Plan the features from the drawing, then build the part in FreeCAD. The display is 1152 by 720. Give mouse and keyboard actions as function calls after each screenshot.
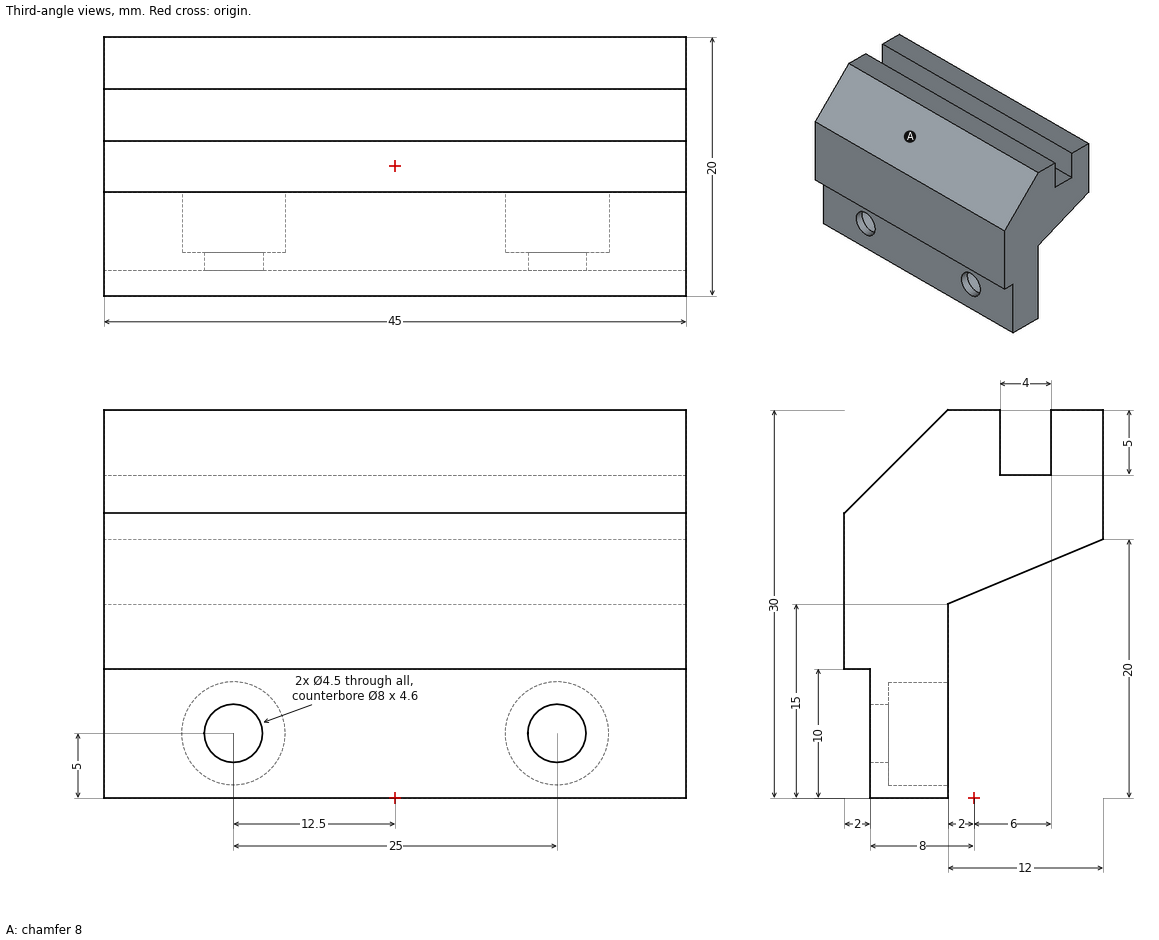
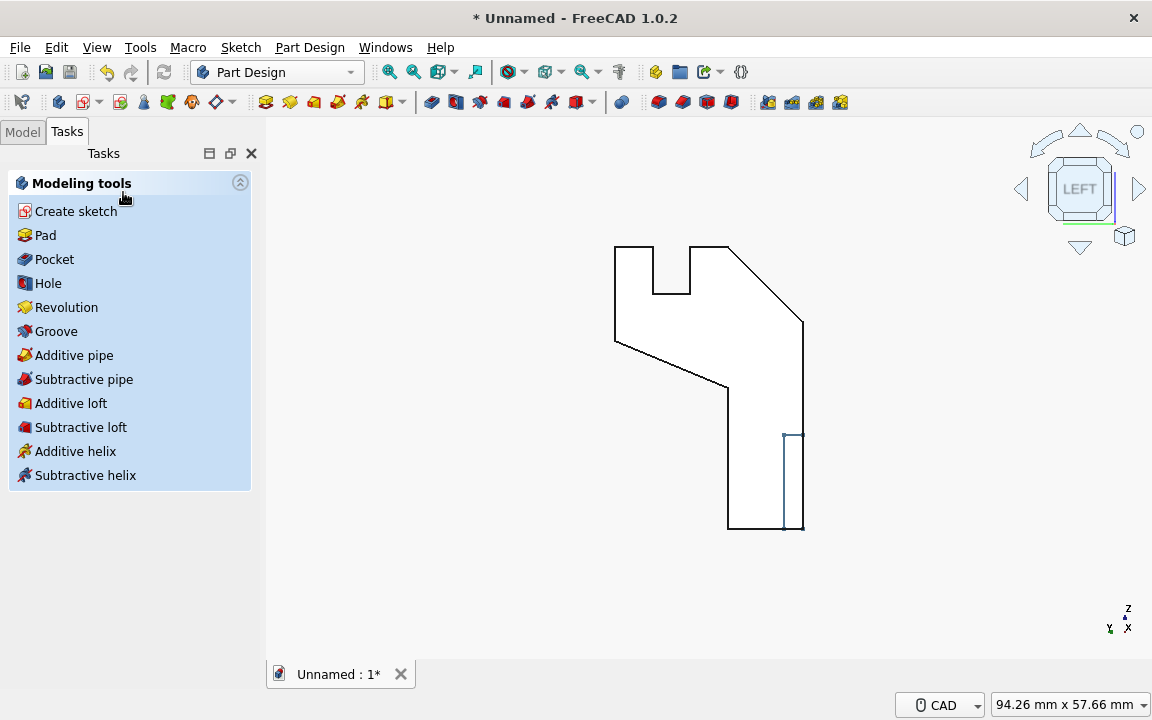
click(432, 102)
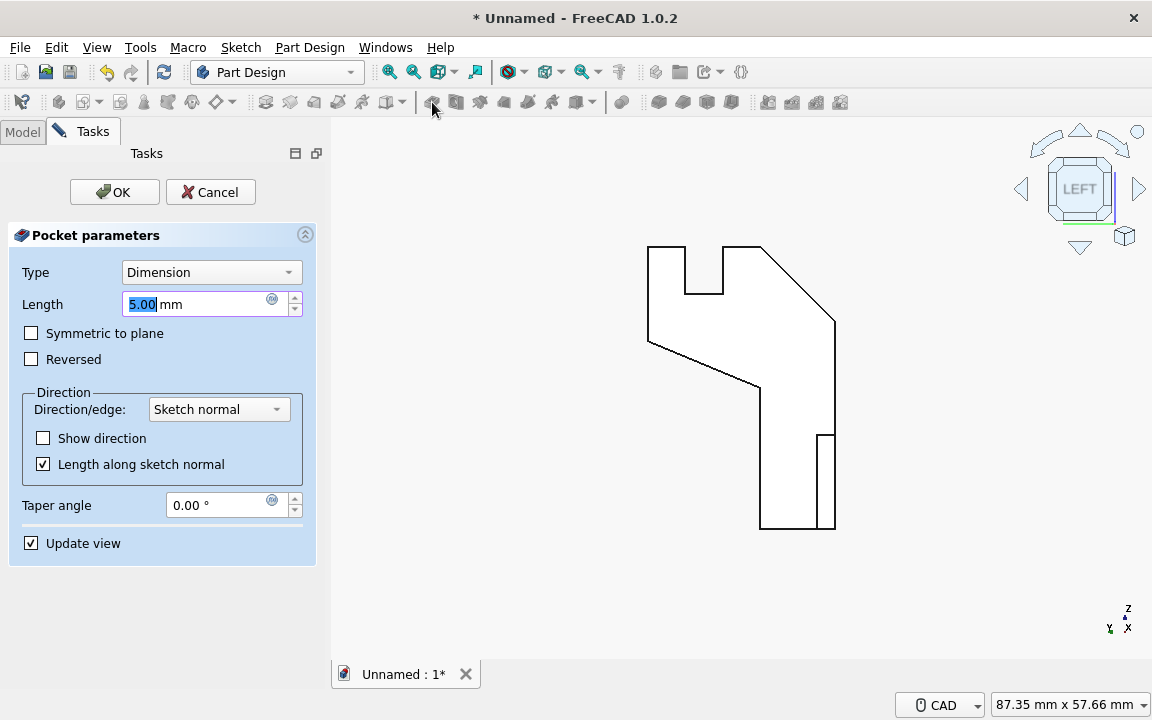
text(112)
key(Tab)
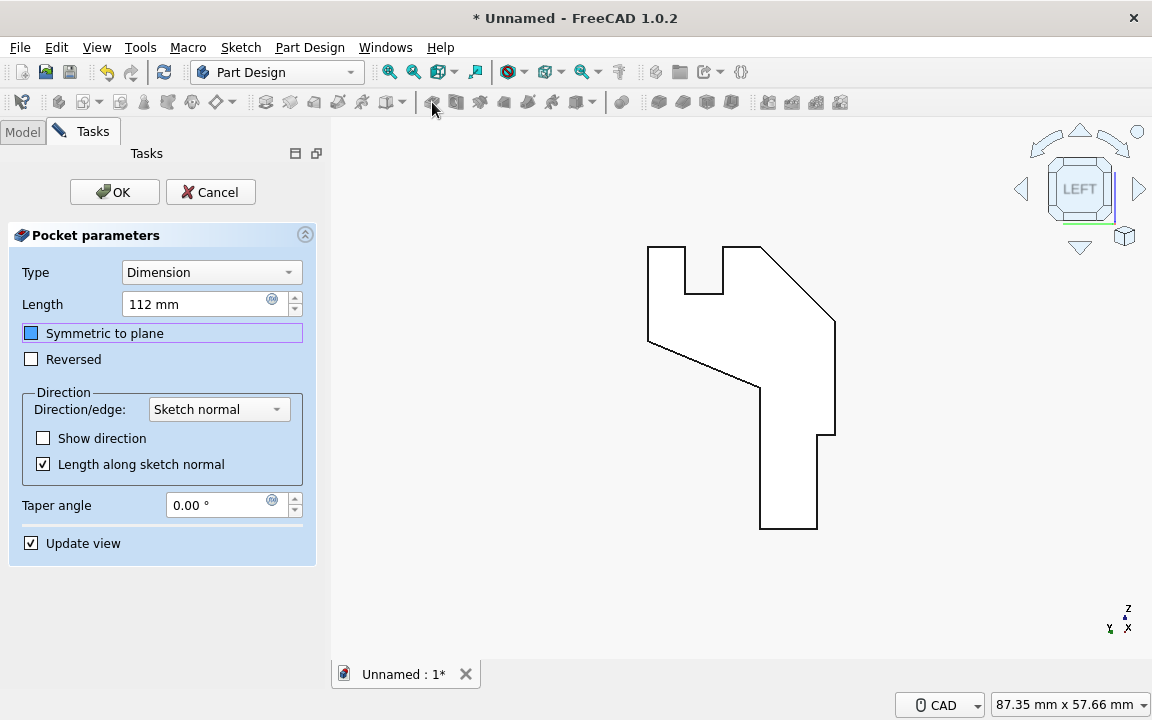
click(30, 333)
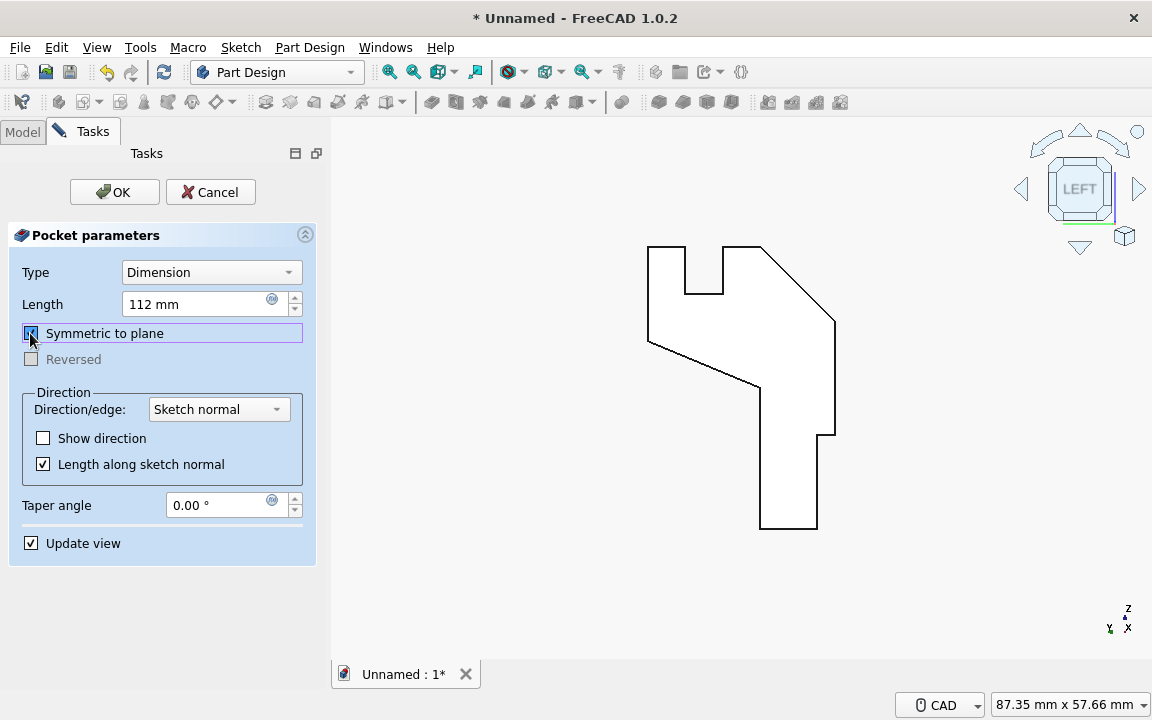
click(115, 192)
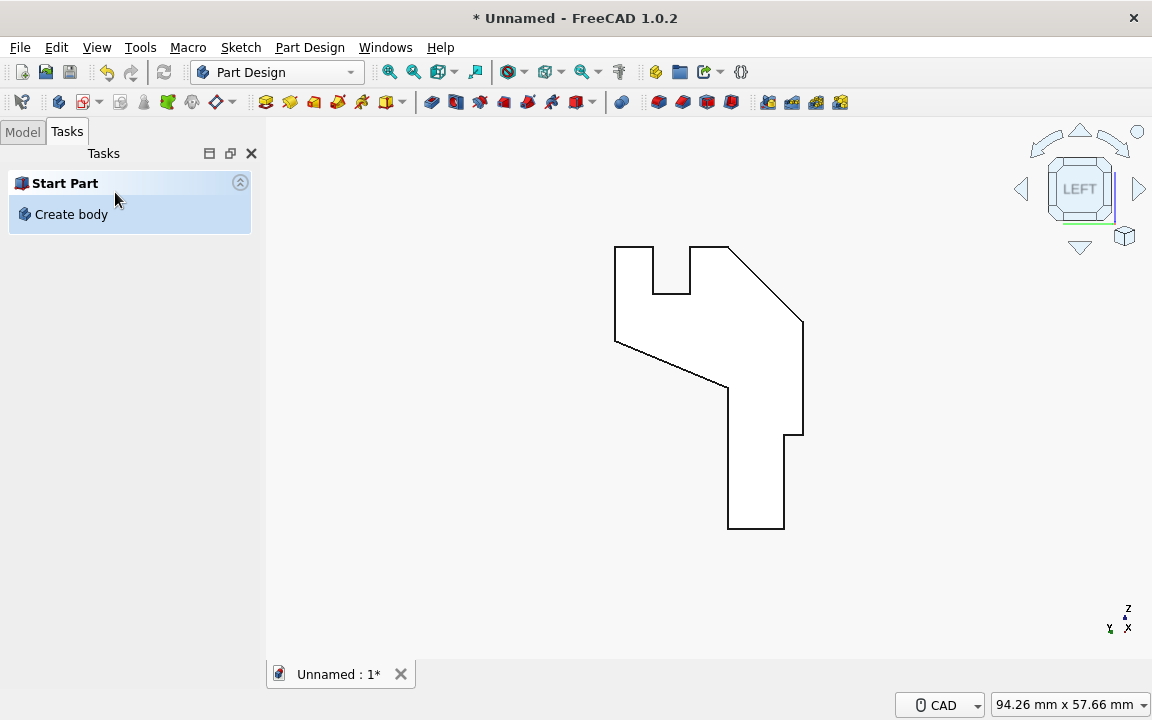
key(0)